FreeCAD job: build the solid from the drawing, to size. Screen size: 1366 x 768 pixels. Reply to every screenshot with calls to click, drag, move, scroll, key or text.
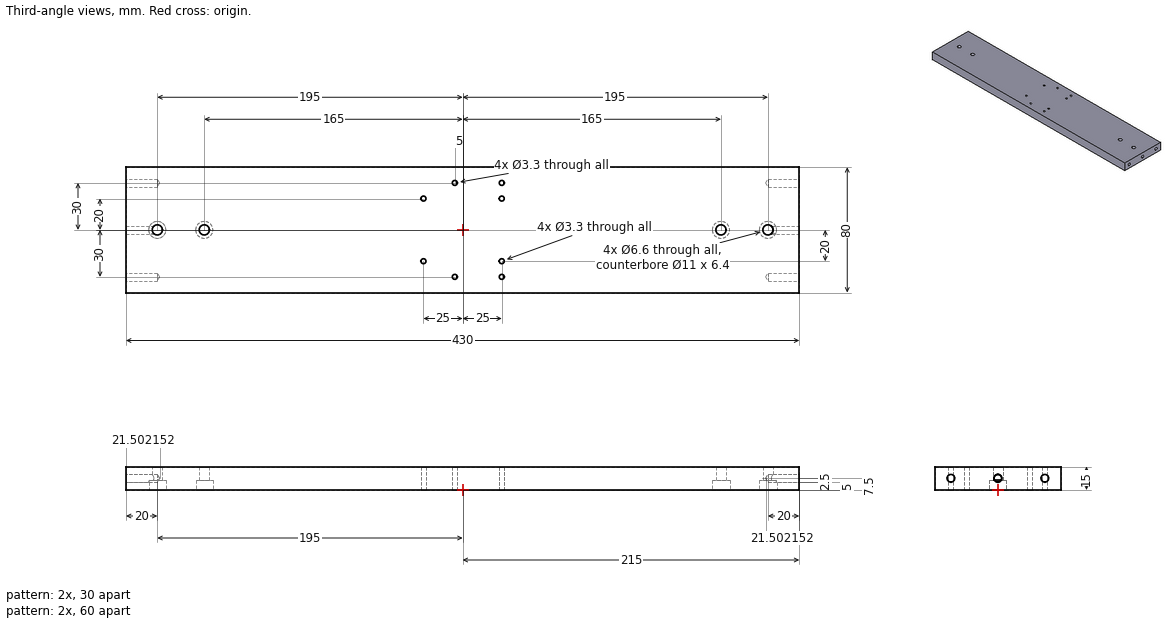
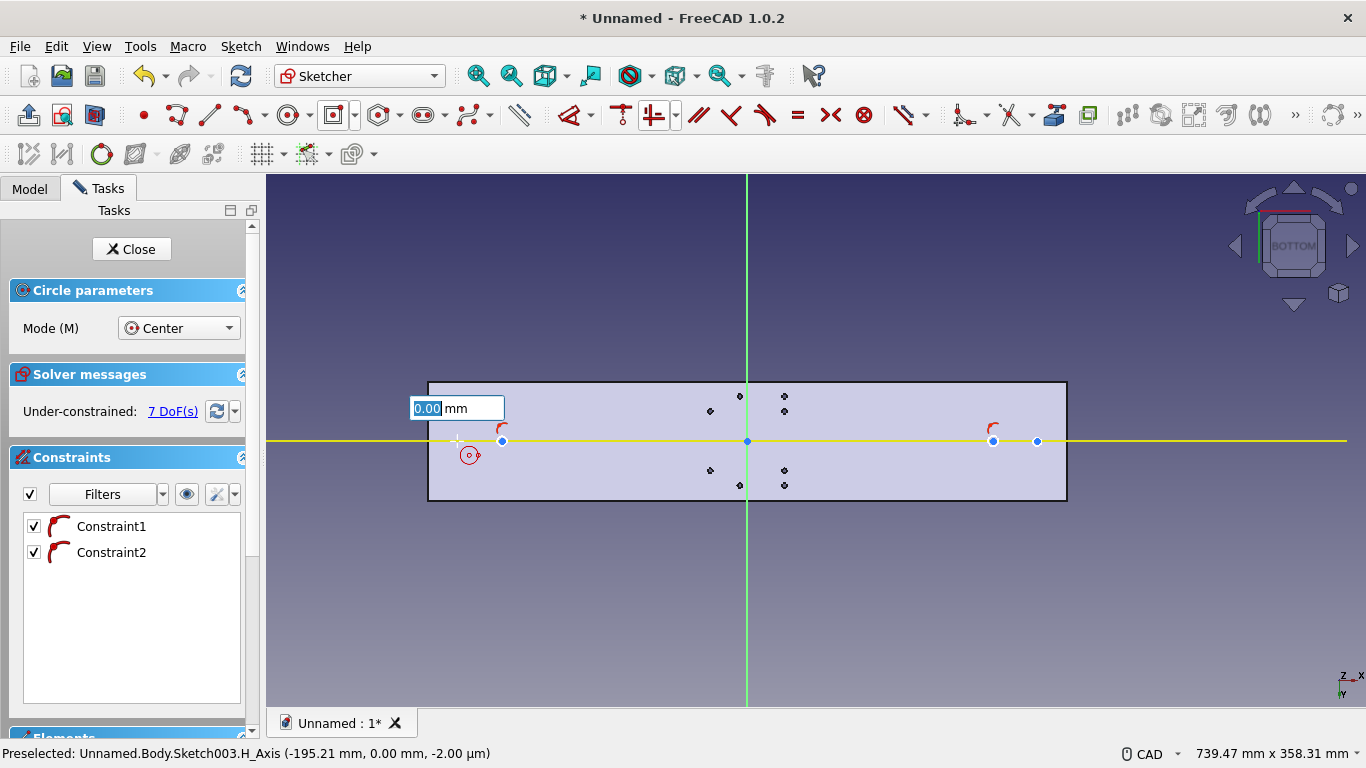
scroll(456, 446, up, 7)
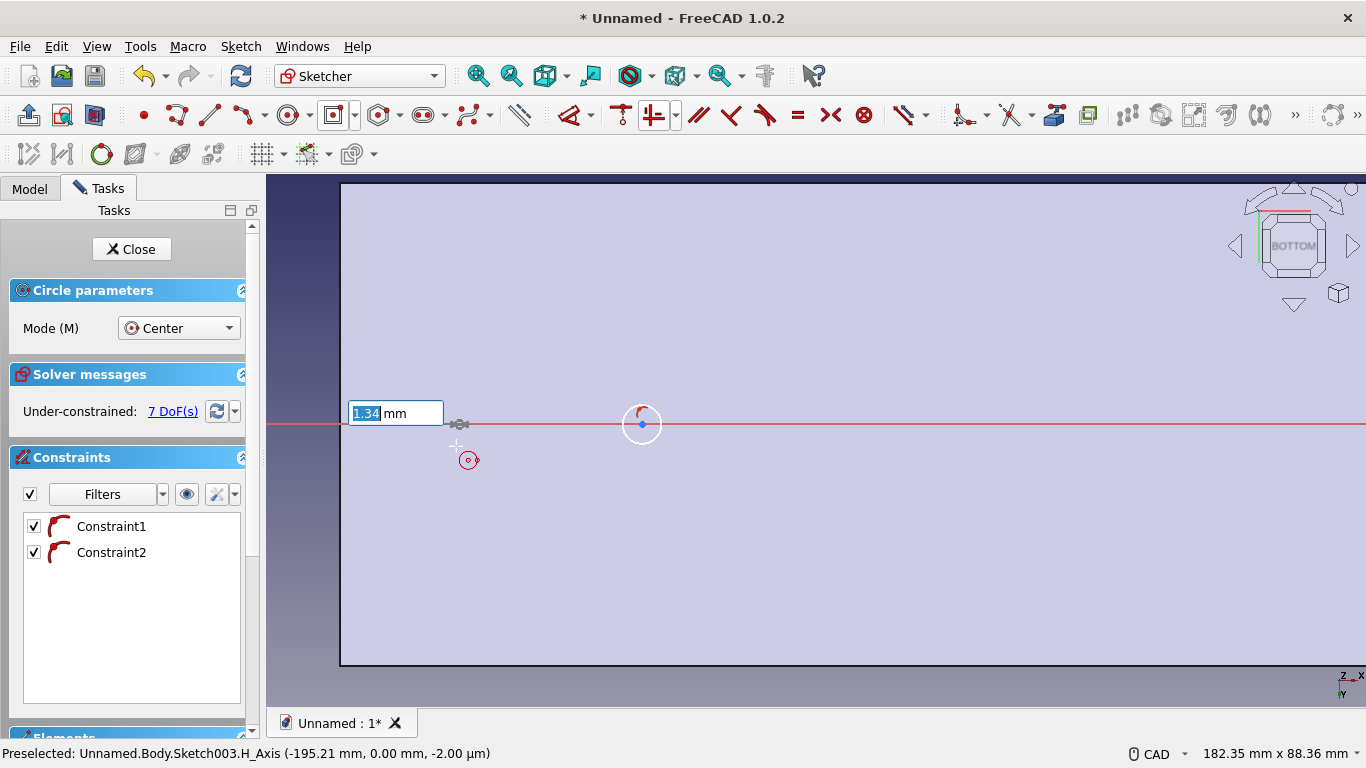
click(454, 443)
key(Escape)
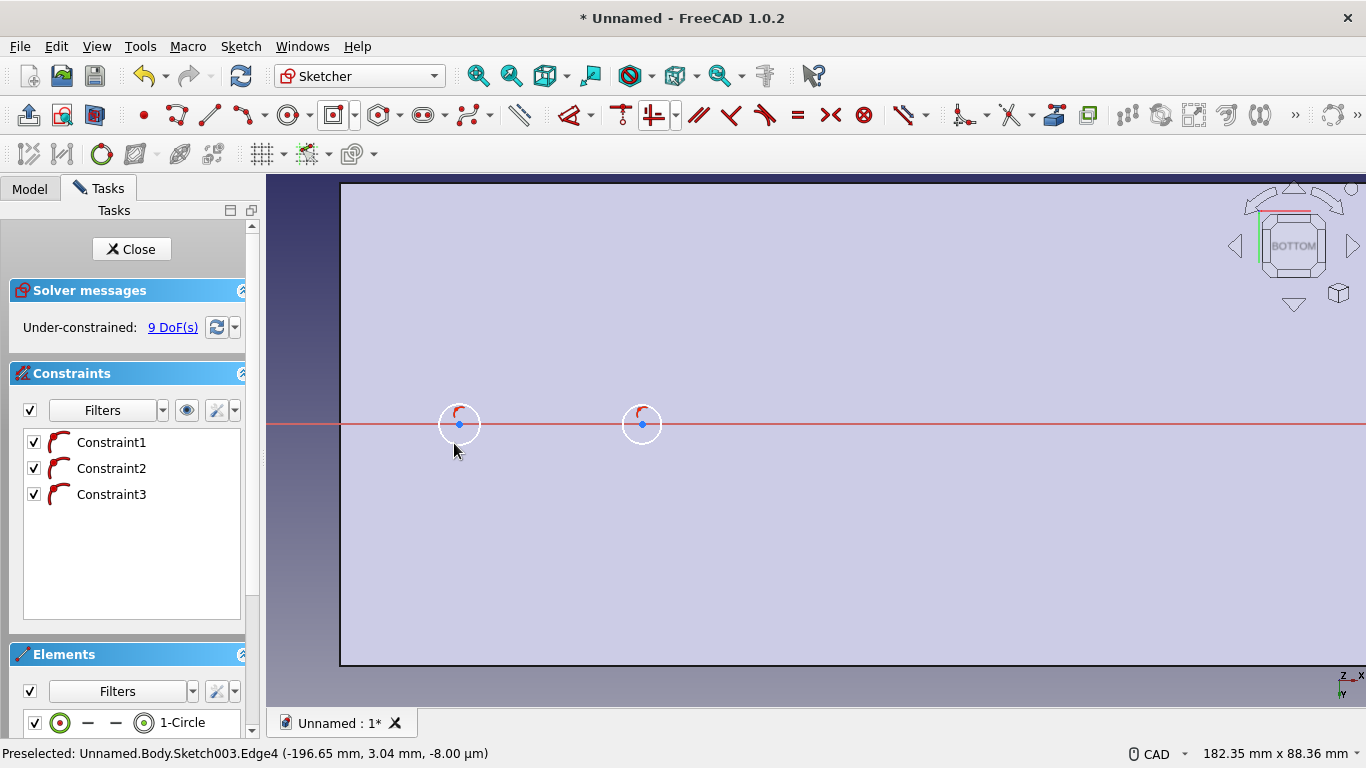
scroll(456, 446, down, 7)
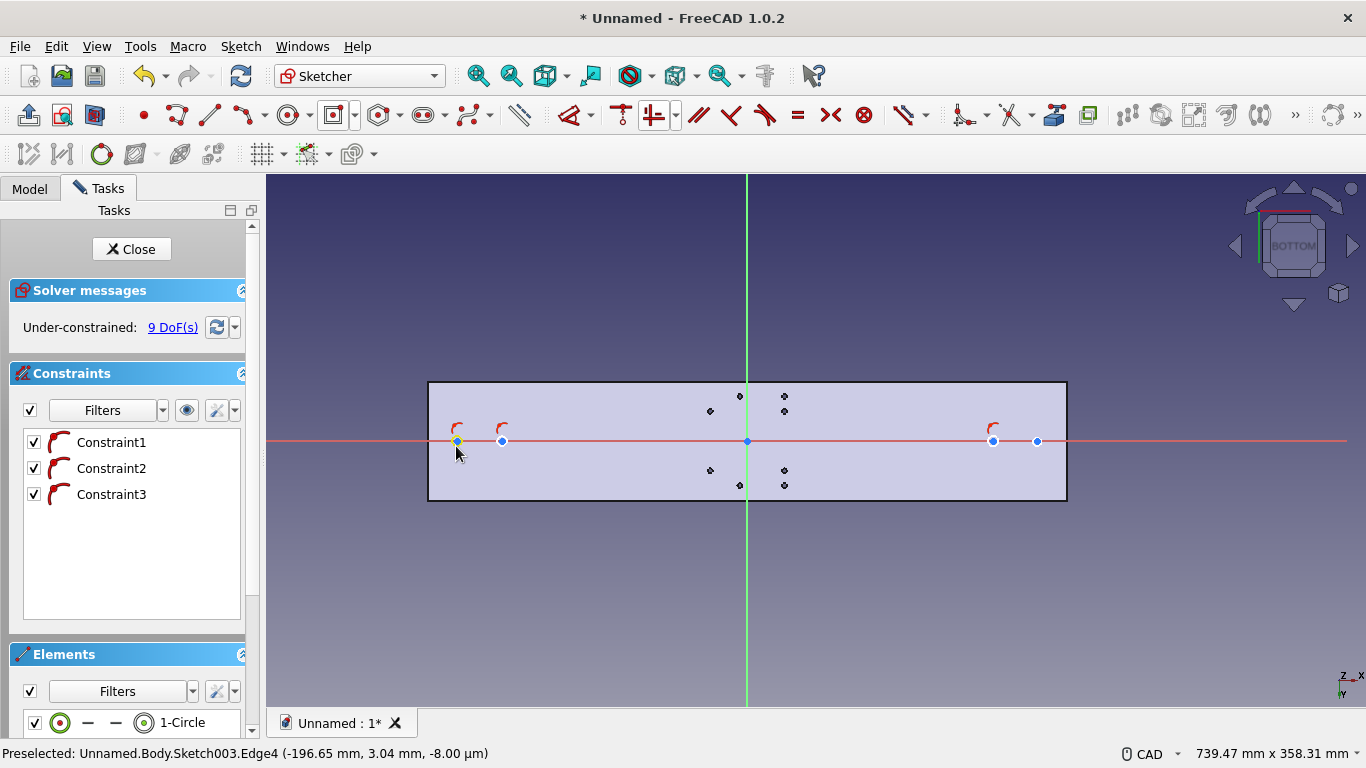
scroll(1034, 445, up, 7)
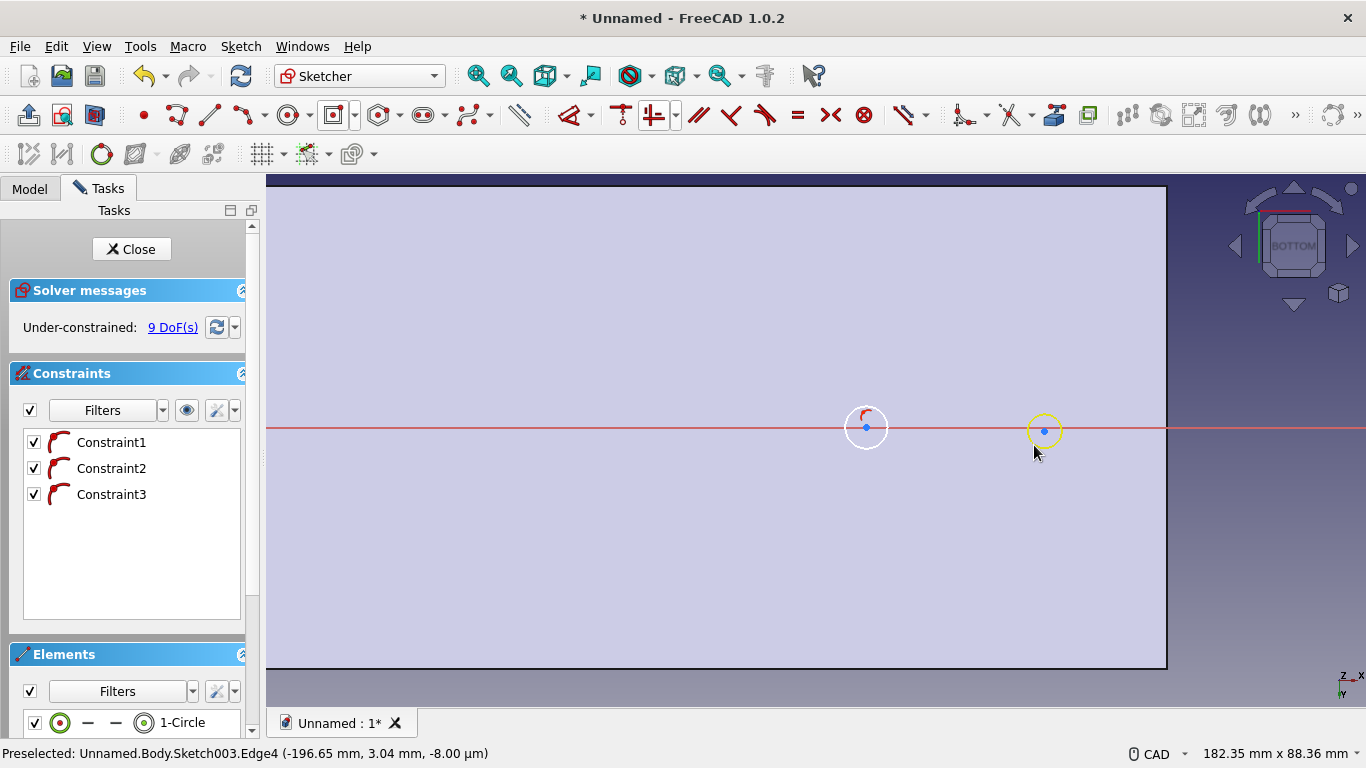
click(1033, 443)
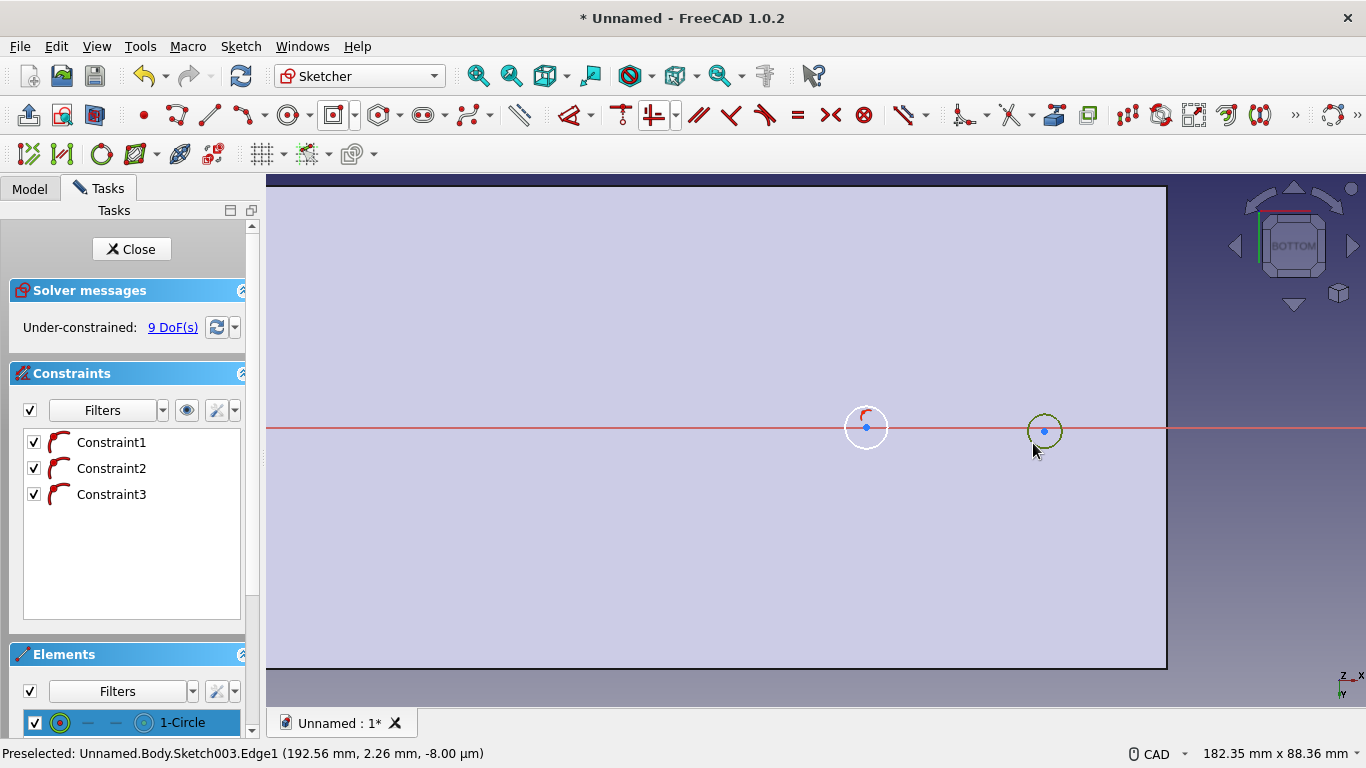
click(881, 413)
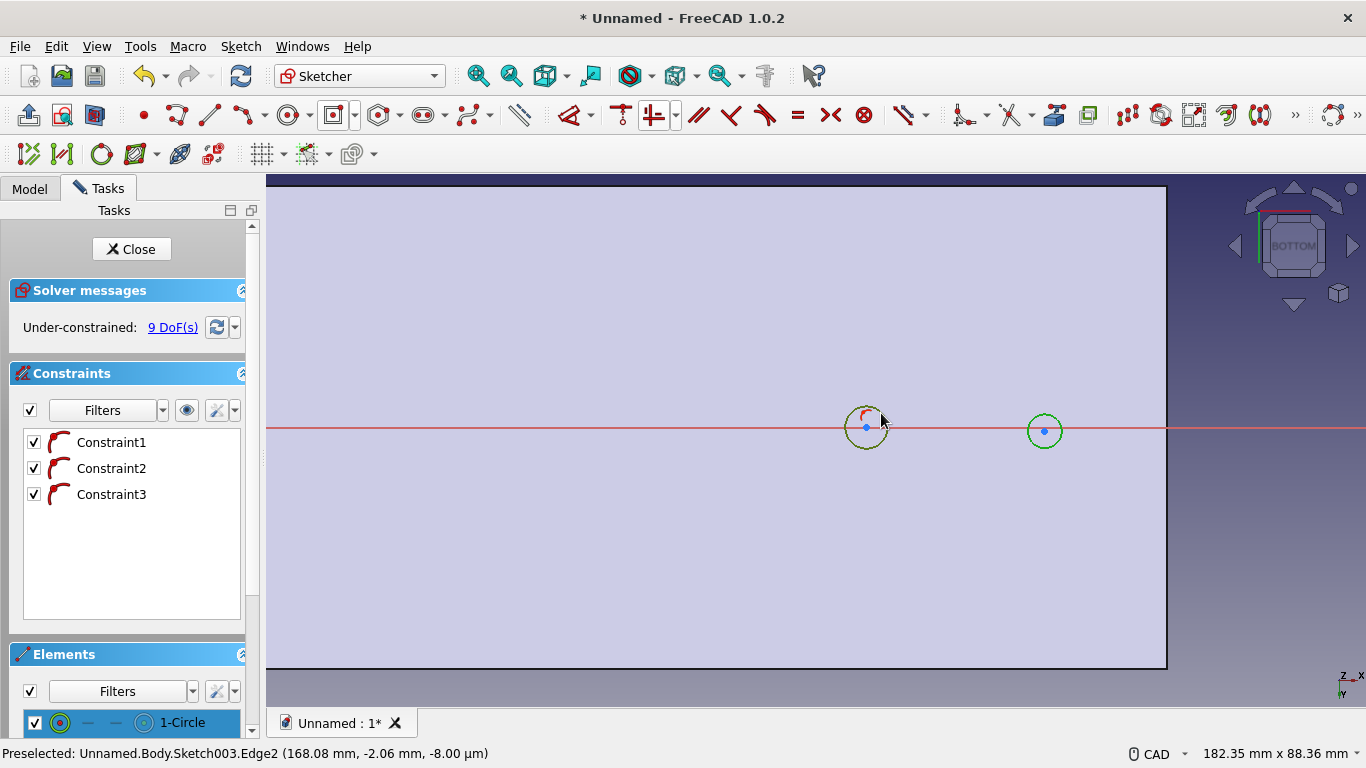
scroll(1035, 445, down, 7)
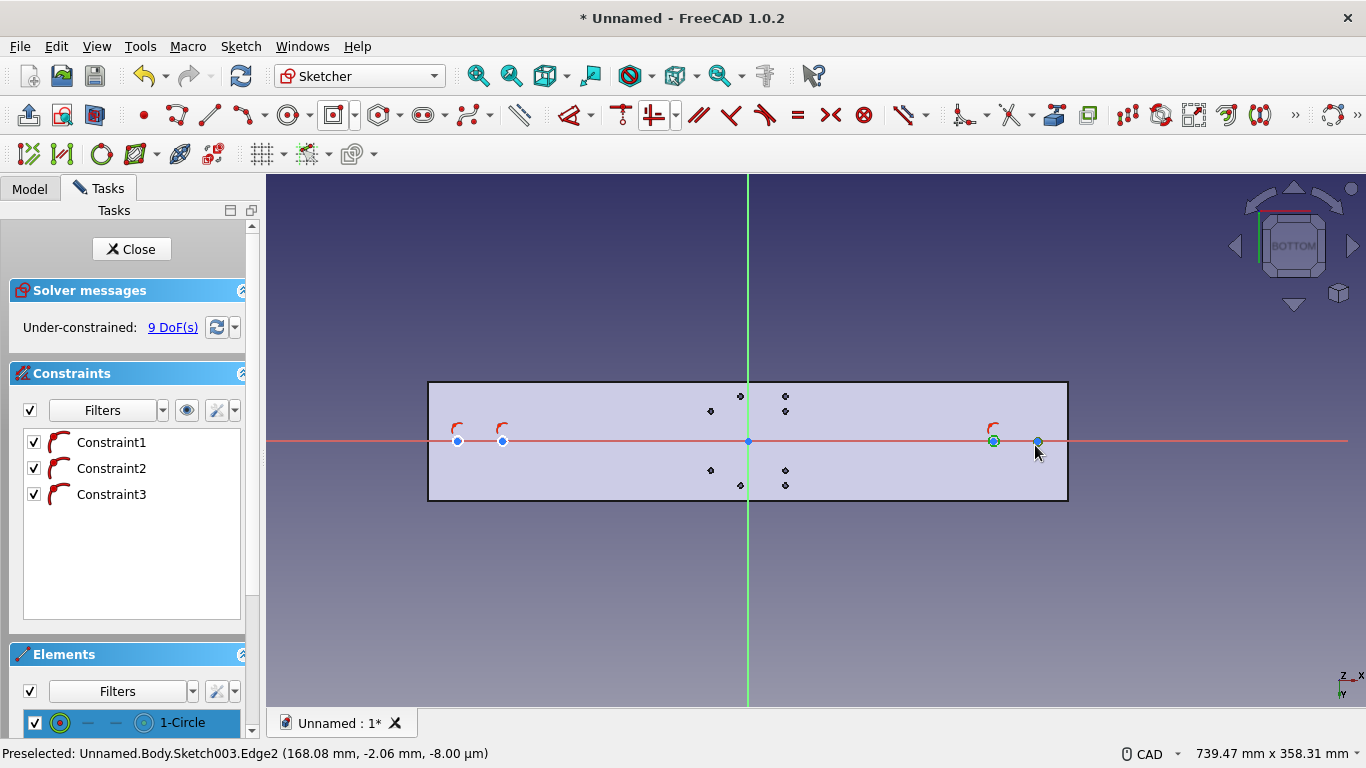
scroll(506, 438, up, 8)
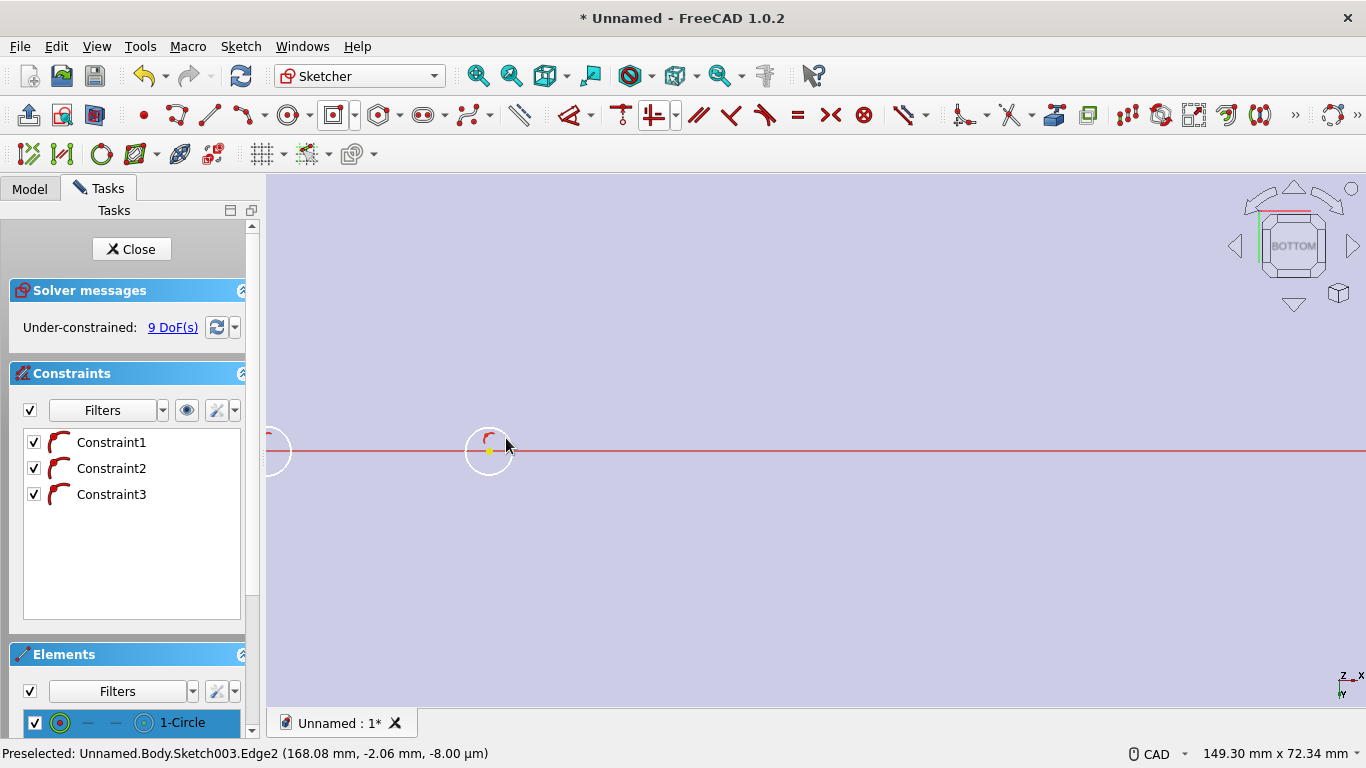
click(506, 435)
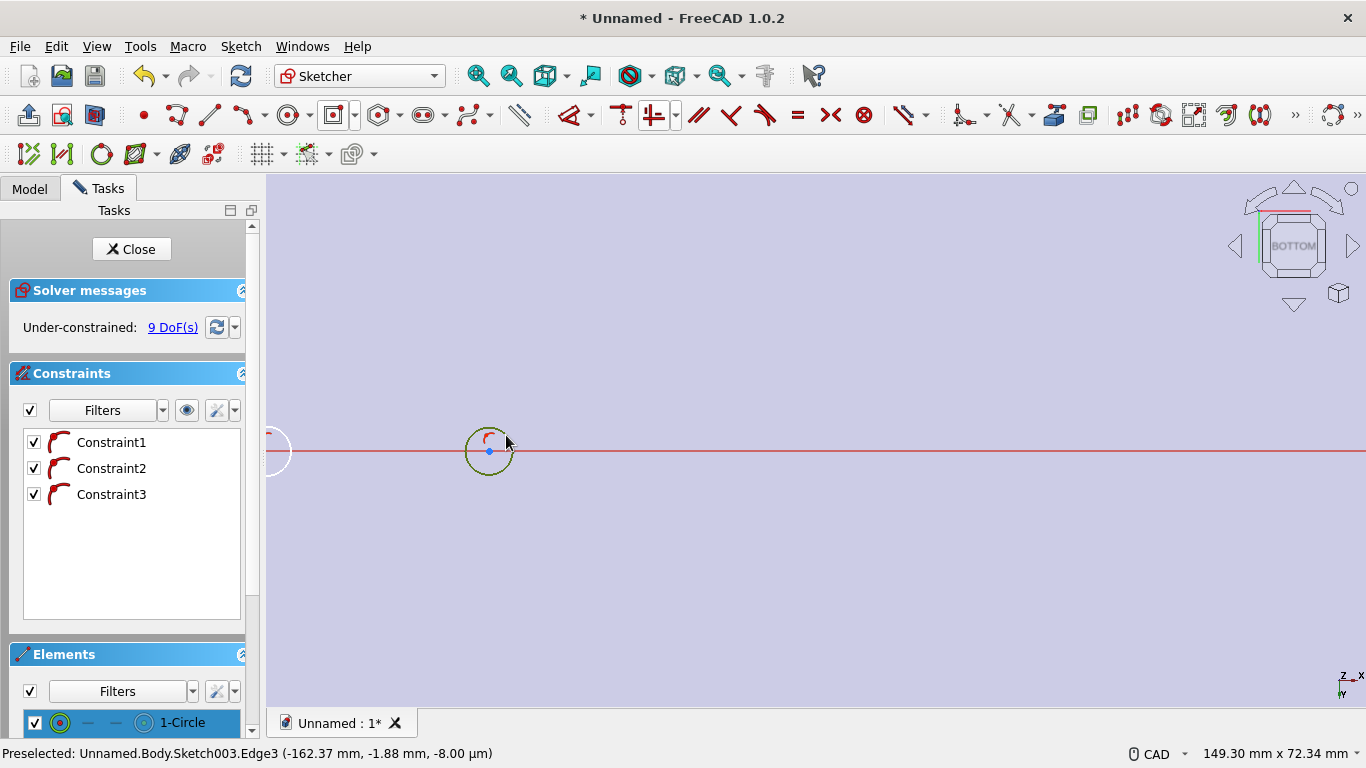
scroll(505, 438, down, 8)